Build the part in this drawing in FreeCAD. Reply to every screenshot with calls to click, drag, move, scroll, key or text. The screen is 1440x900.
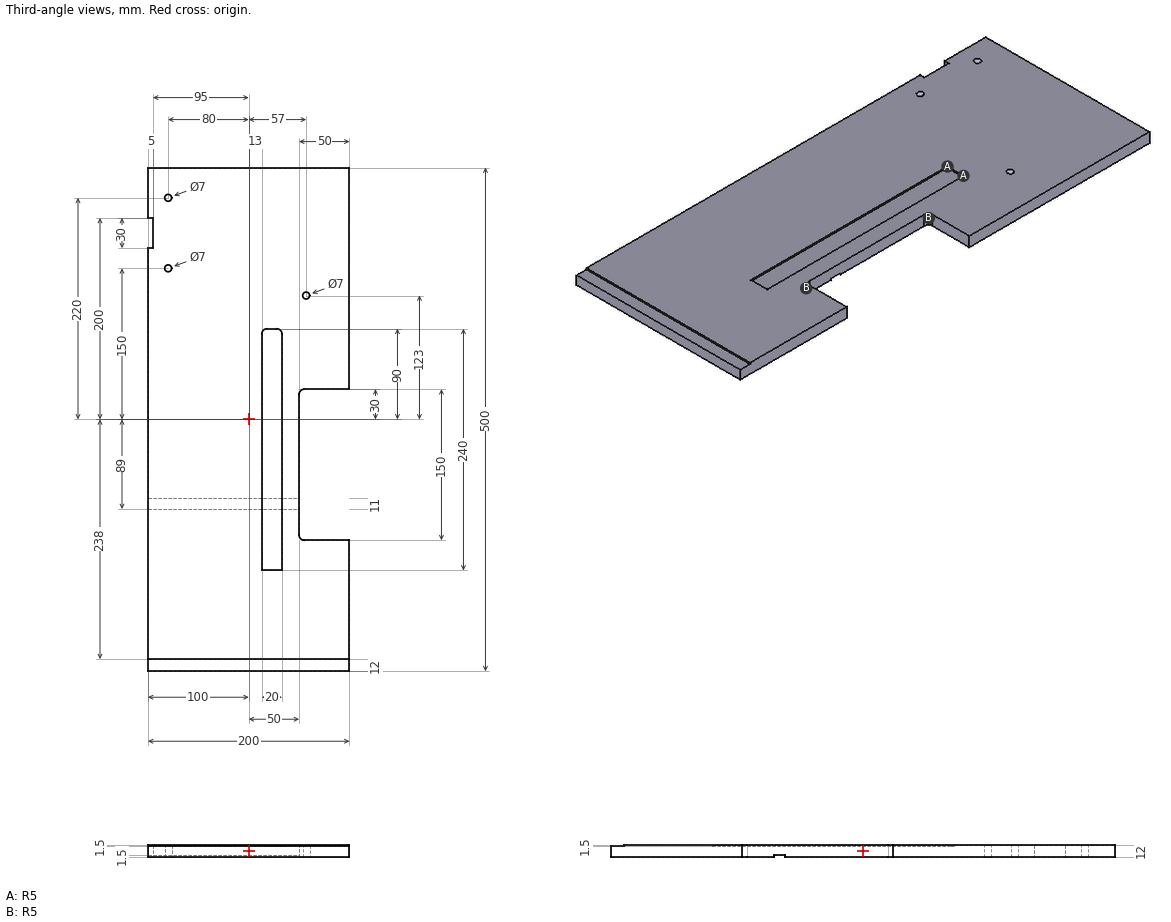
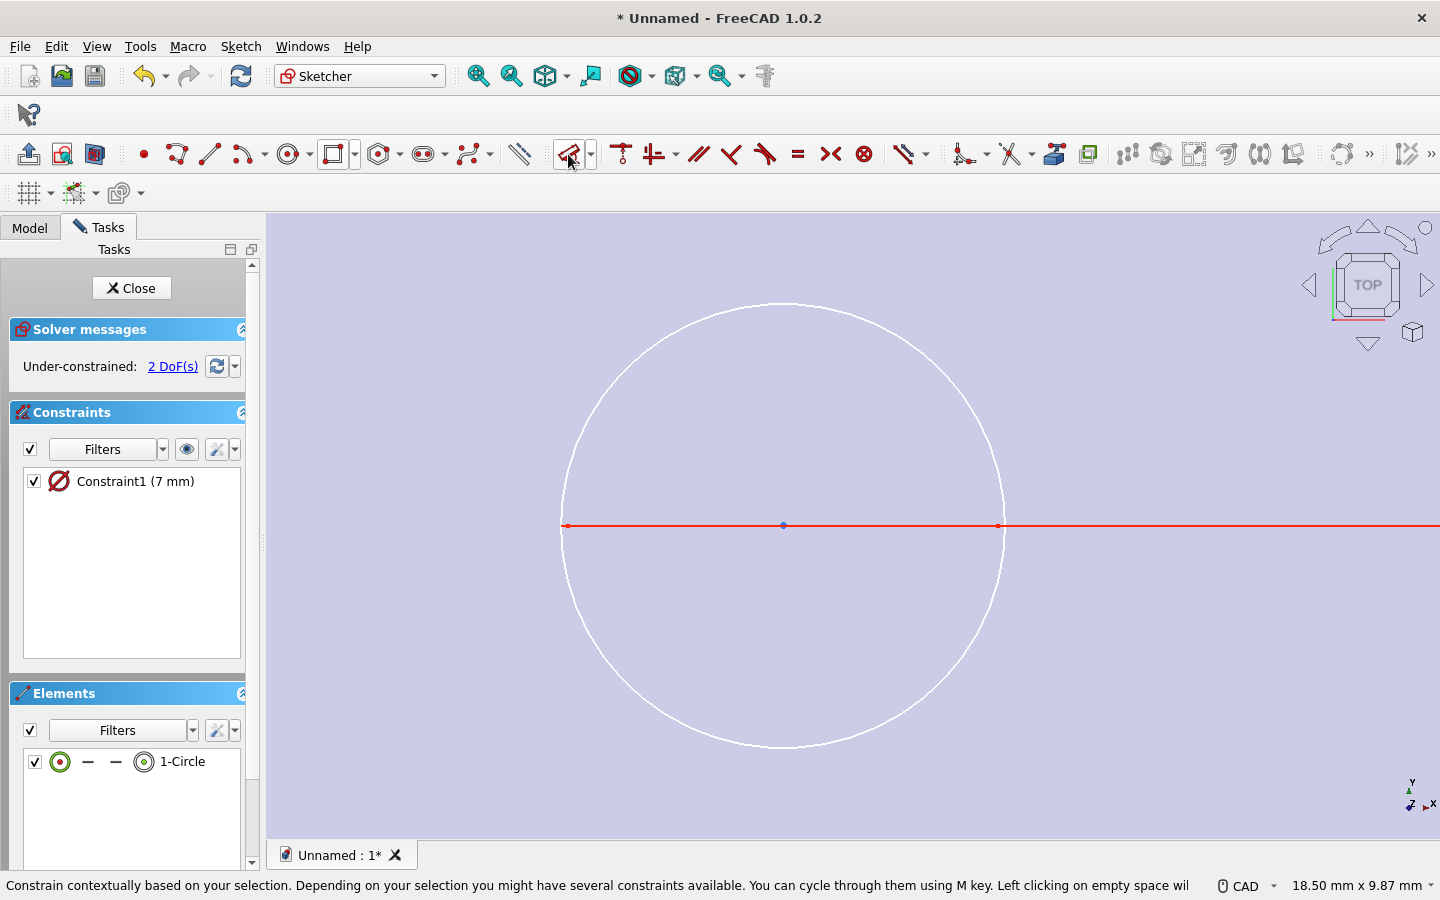
click(783, 526)
click(539, 492)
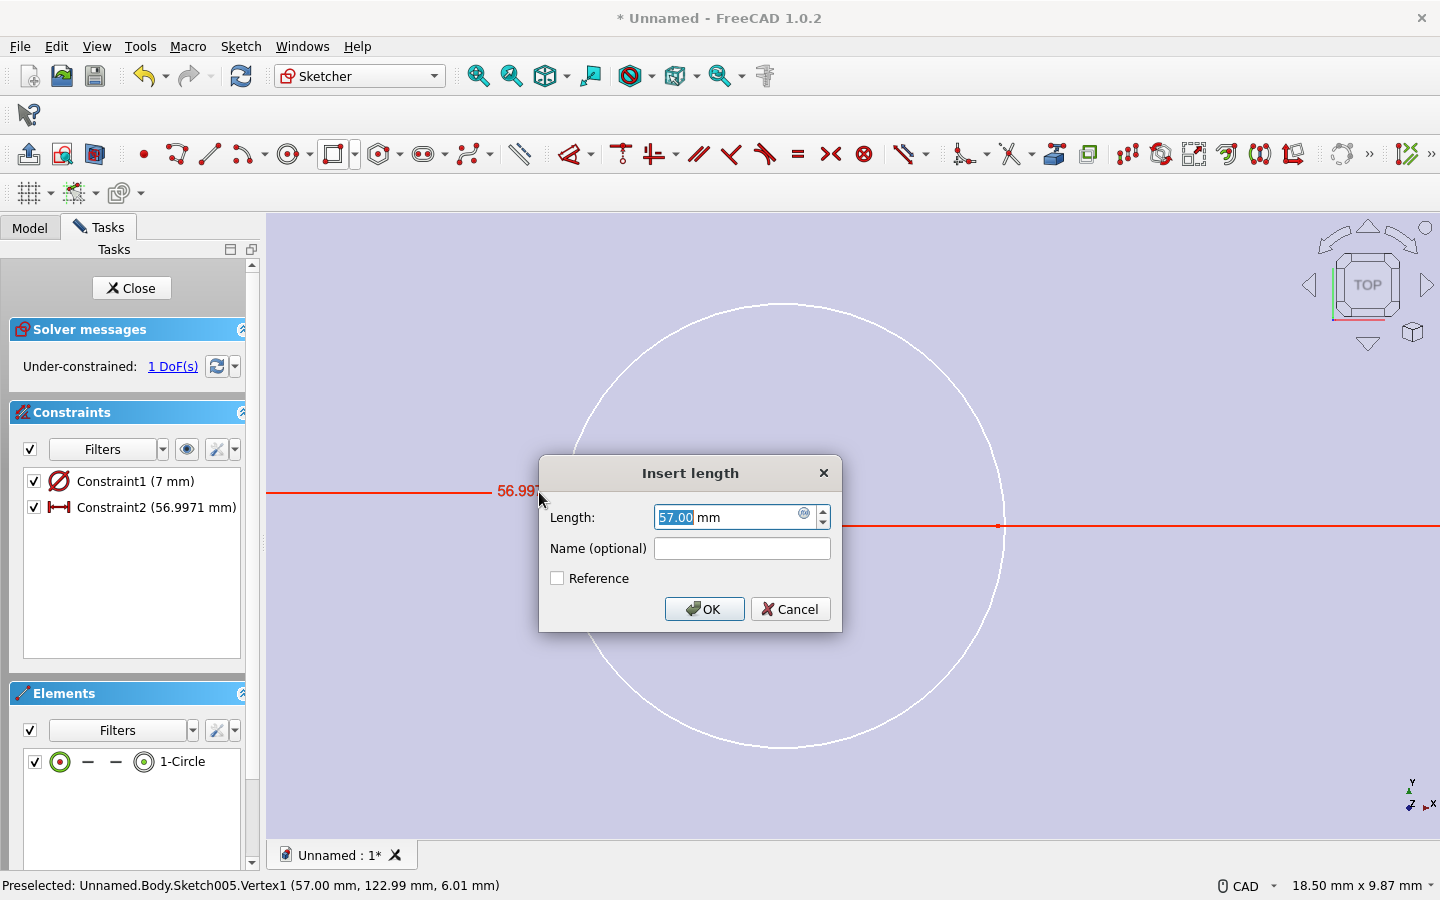
text(57)
key(Return)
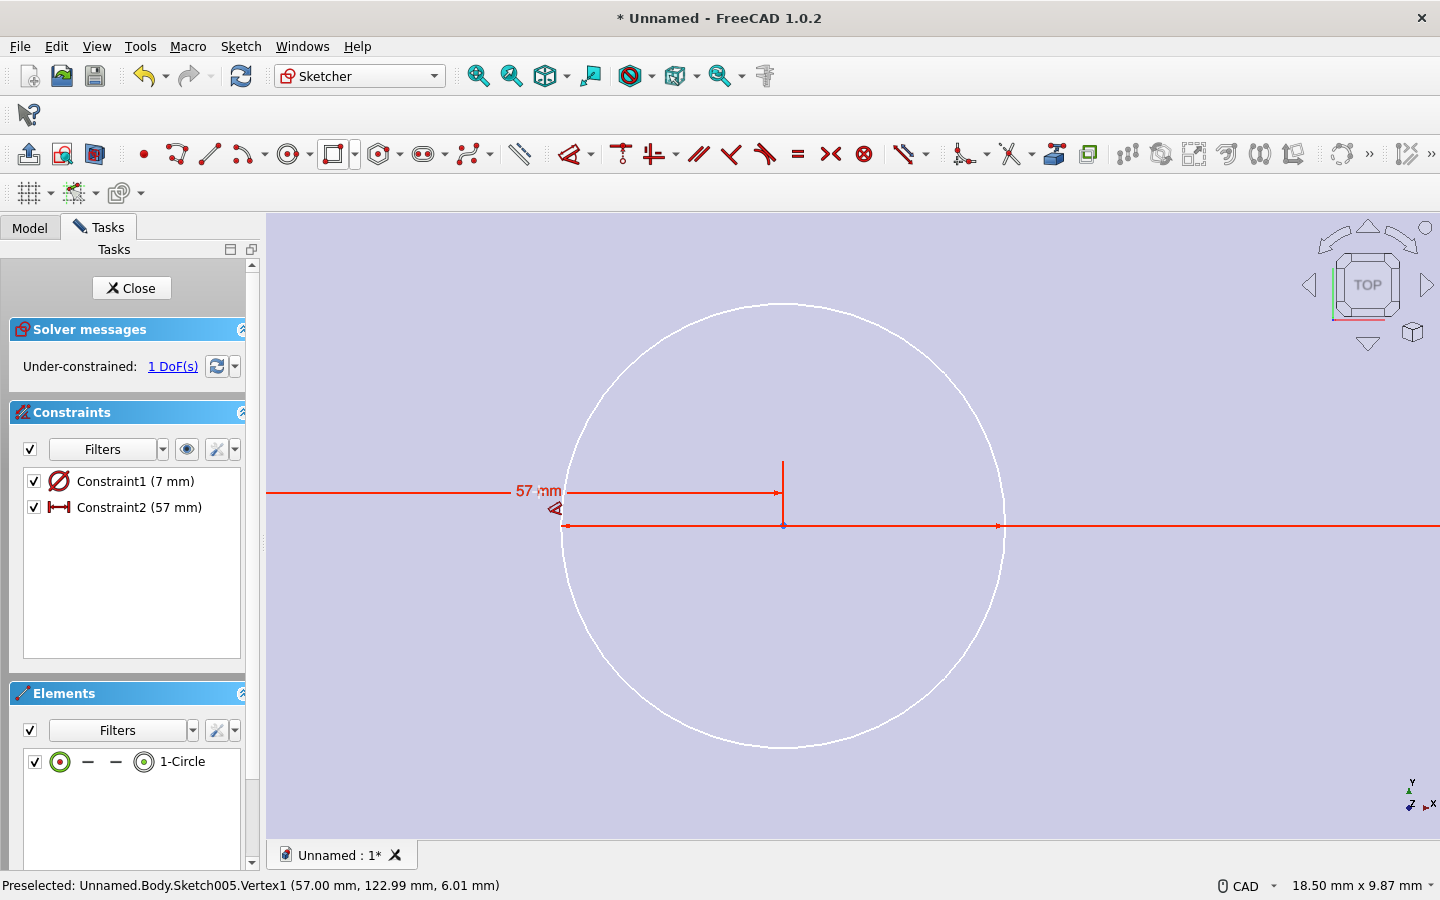
click(783, 526)
click(817, 669)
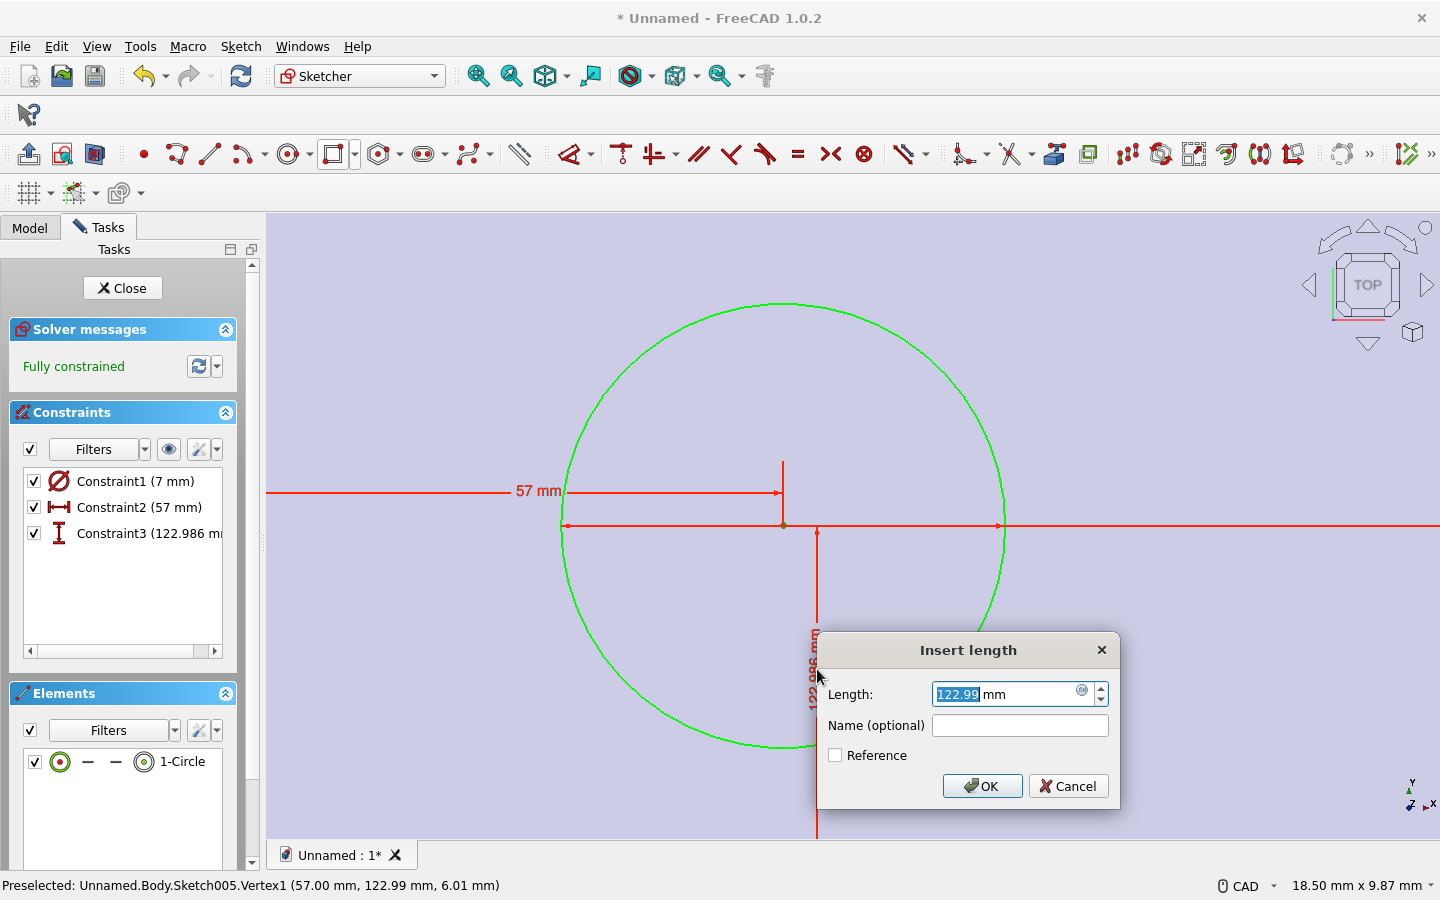
text(123)
key(Return)
key(Escape)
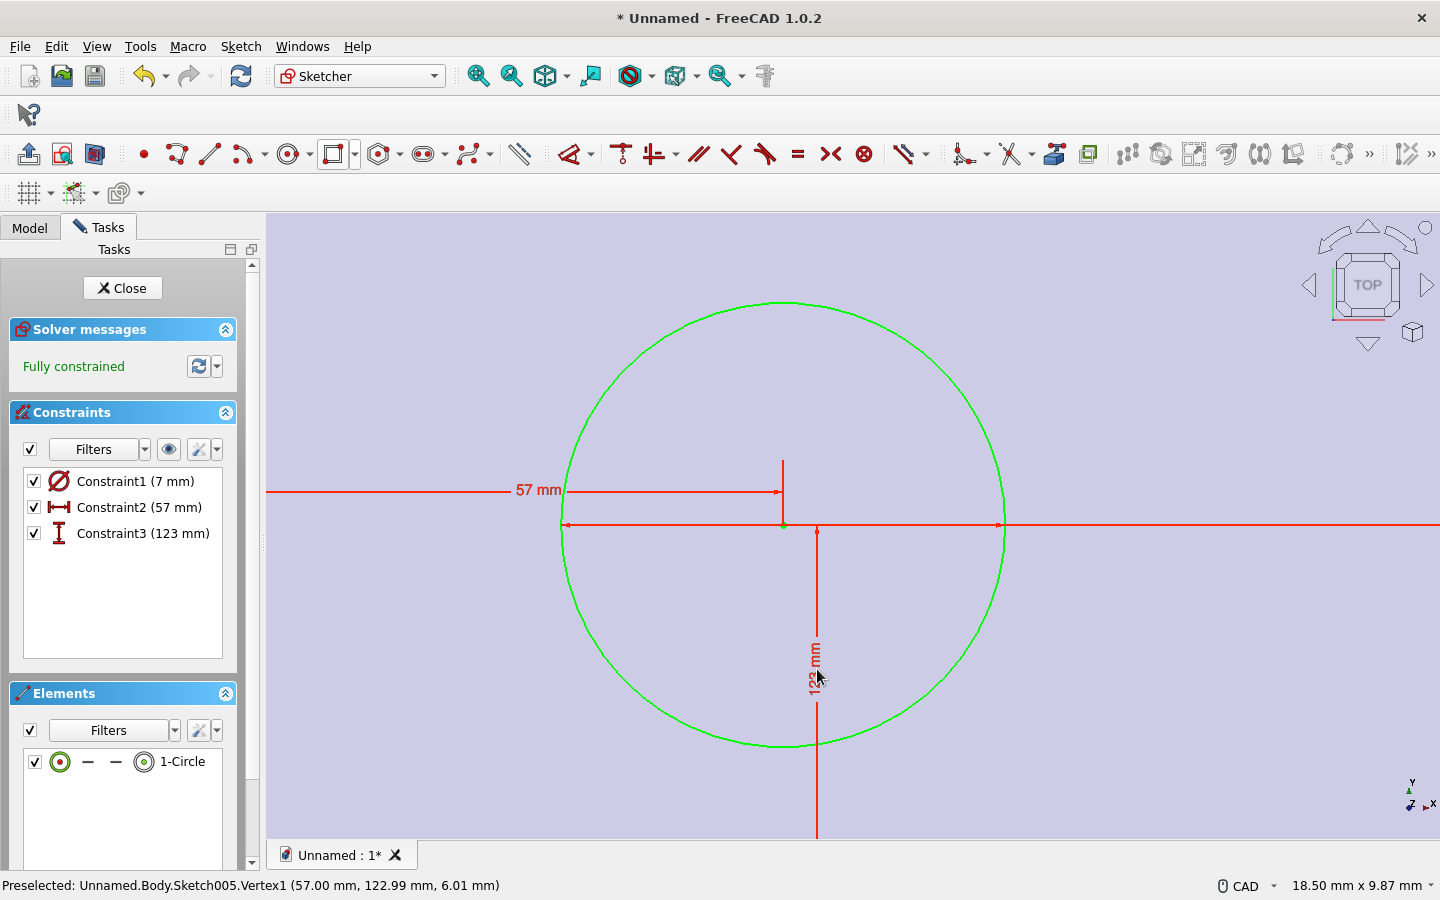
click(123, 288)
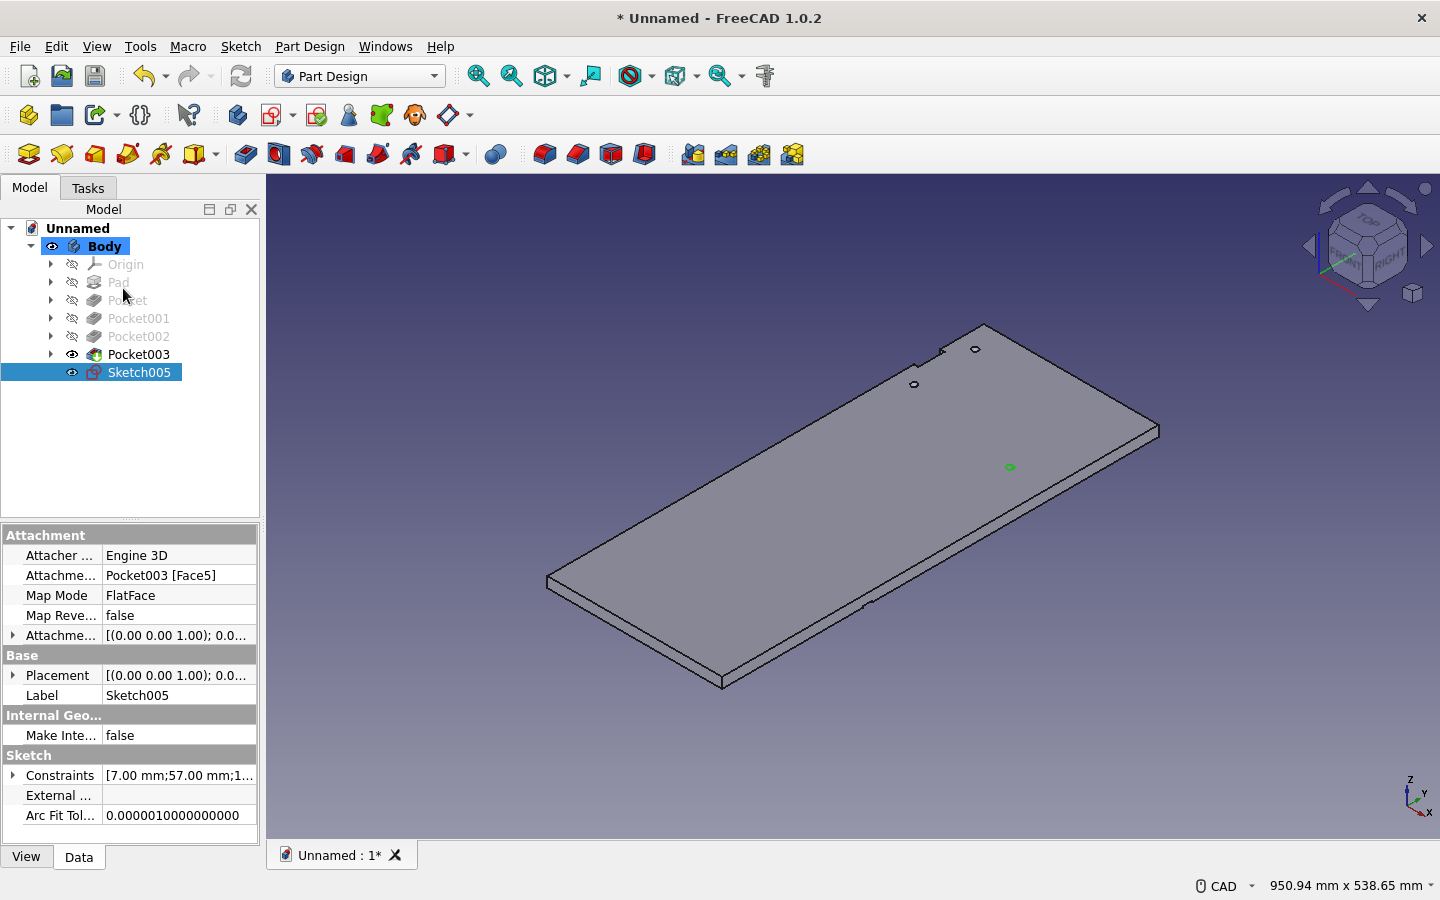
click(246, 154)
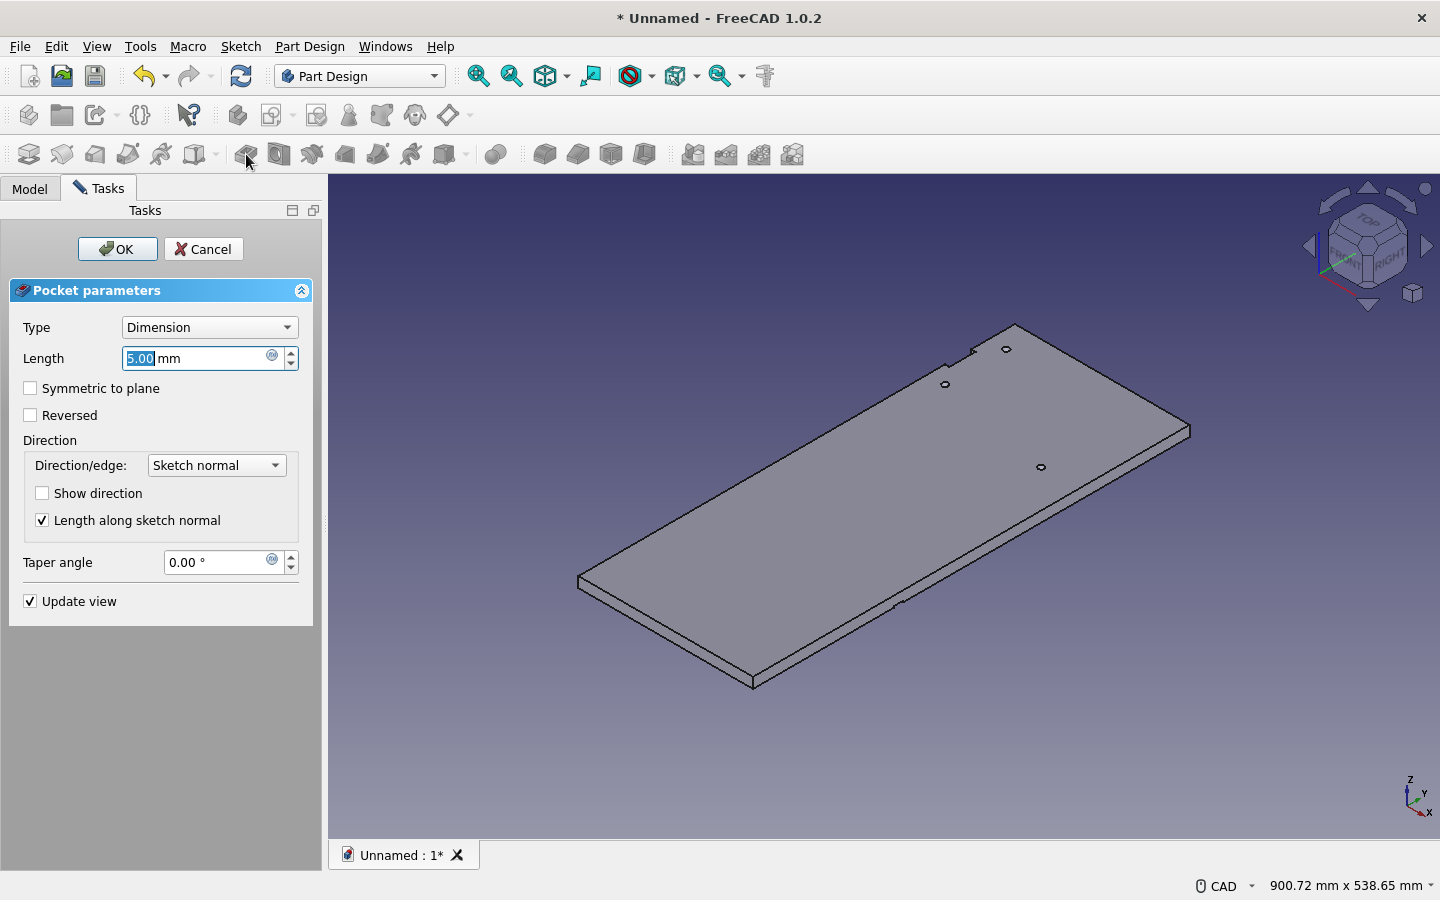
click(210, 328)